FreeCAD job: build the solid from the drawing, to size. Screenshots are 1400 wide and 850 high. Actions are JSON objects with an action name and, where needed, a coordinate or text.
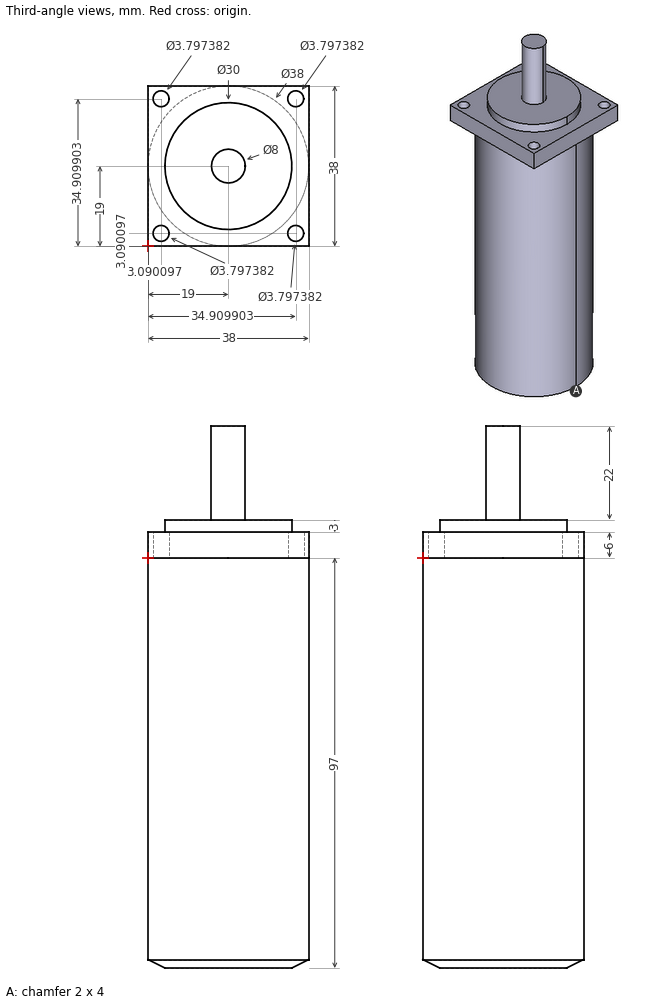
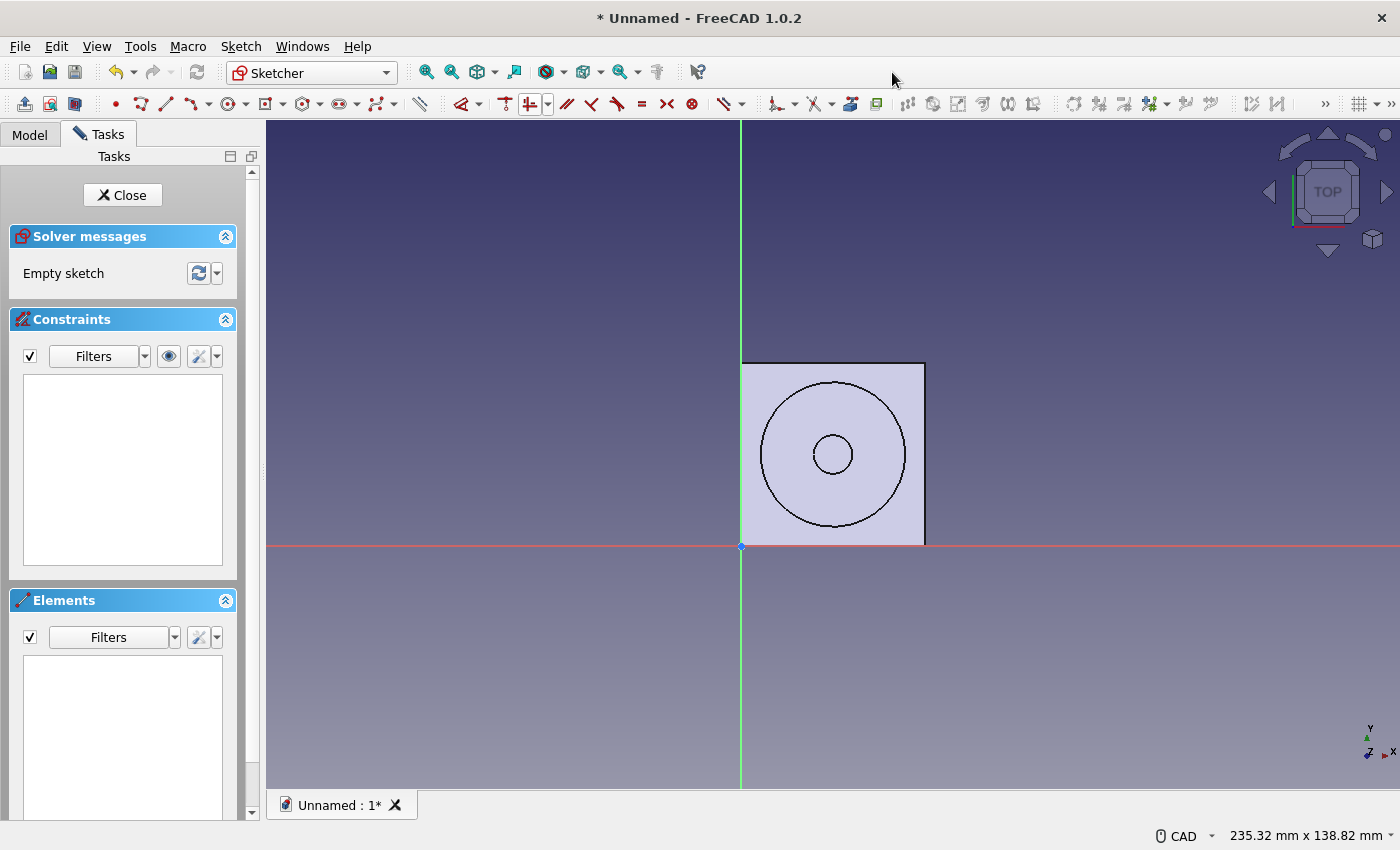
{"action": "scroll", "coordinate": [756, 374], "scroll_direction": "up", "scroll_amount": 15}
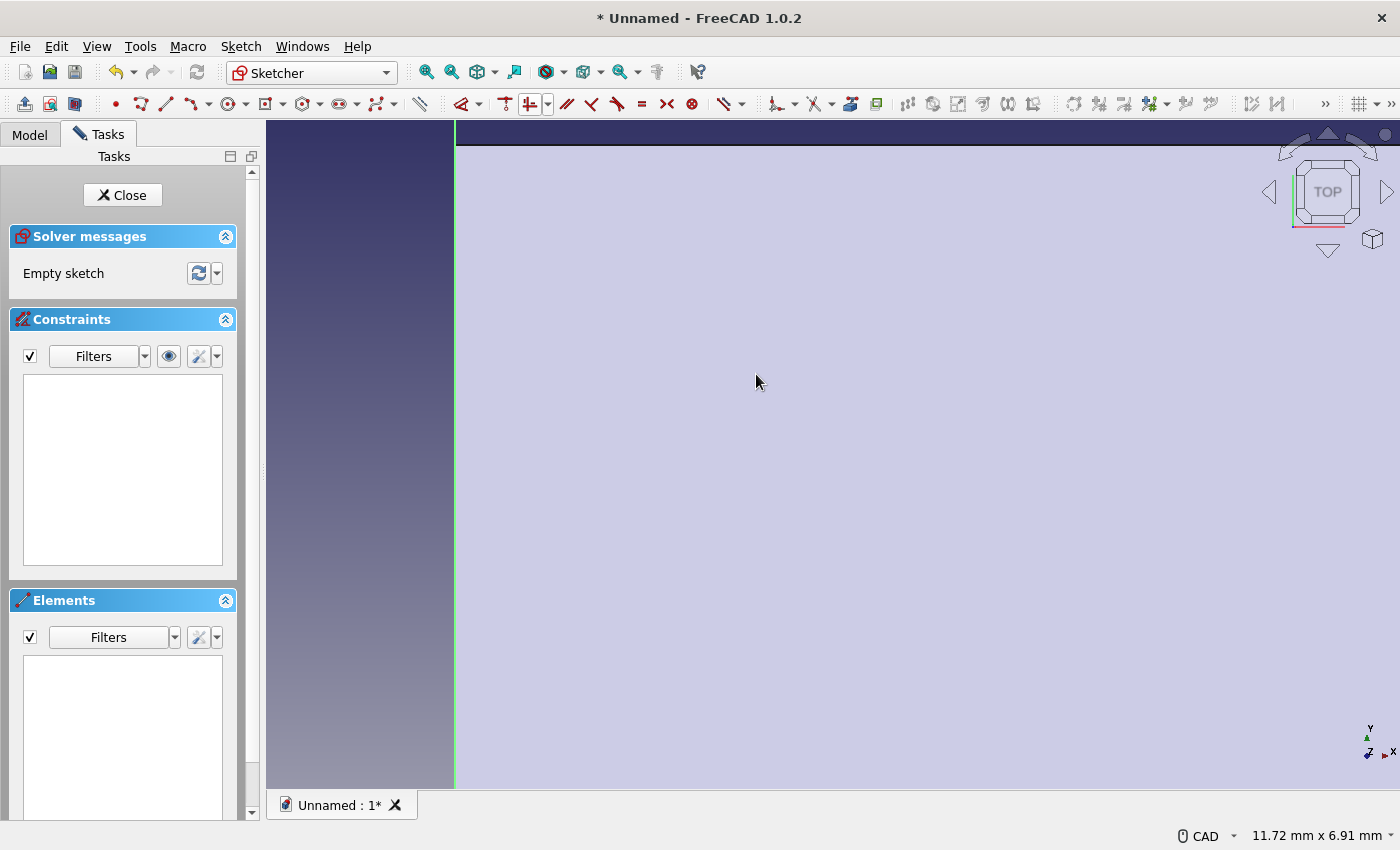
{"action": "key", "text": "g c"}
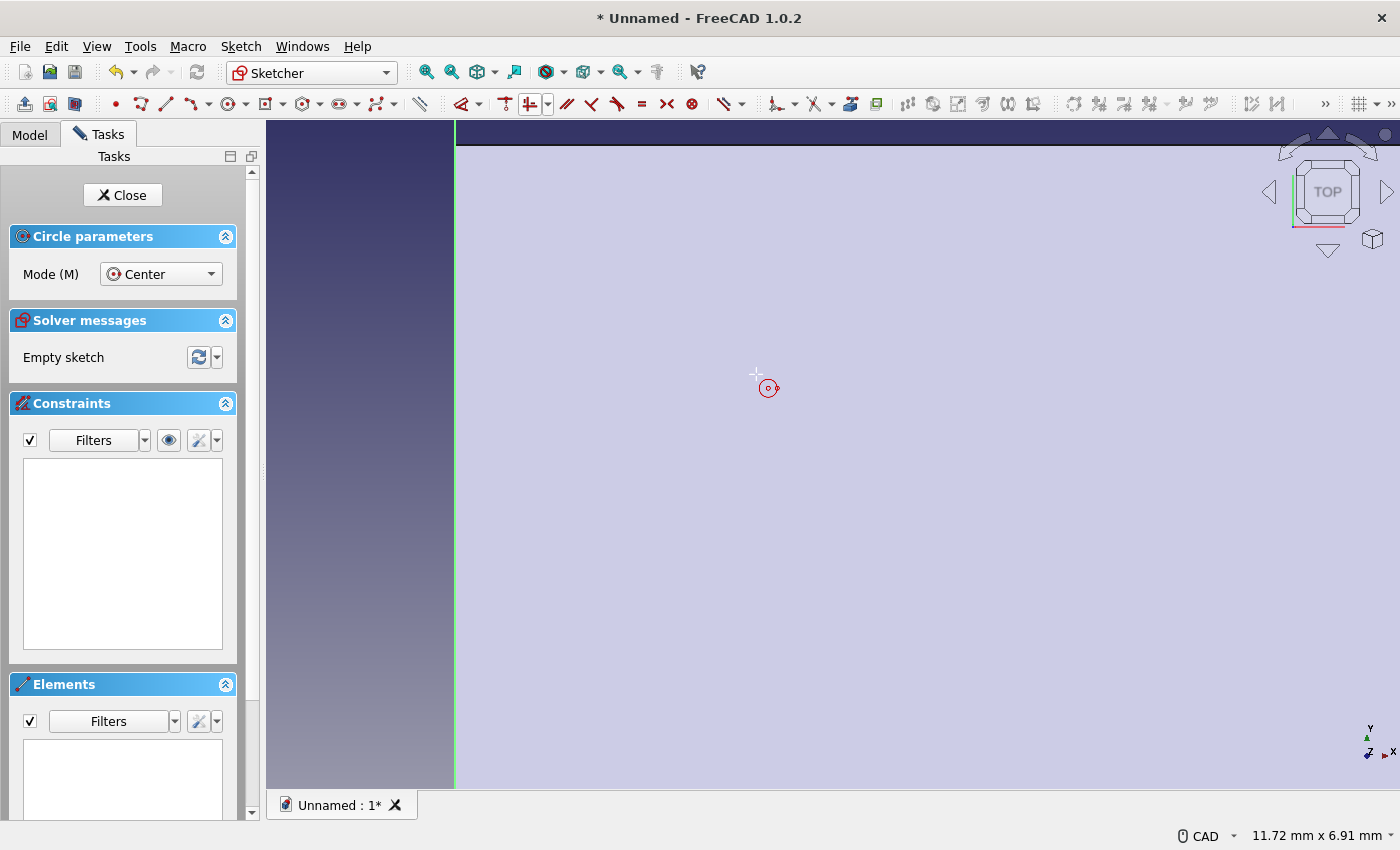
{"action": "left_click", "coordinate": [754, 444]}
{"action": "mouse_move", "coordinate": [884, 314]}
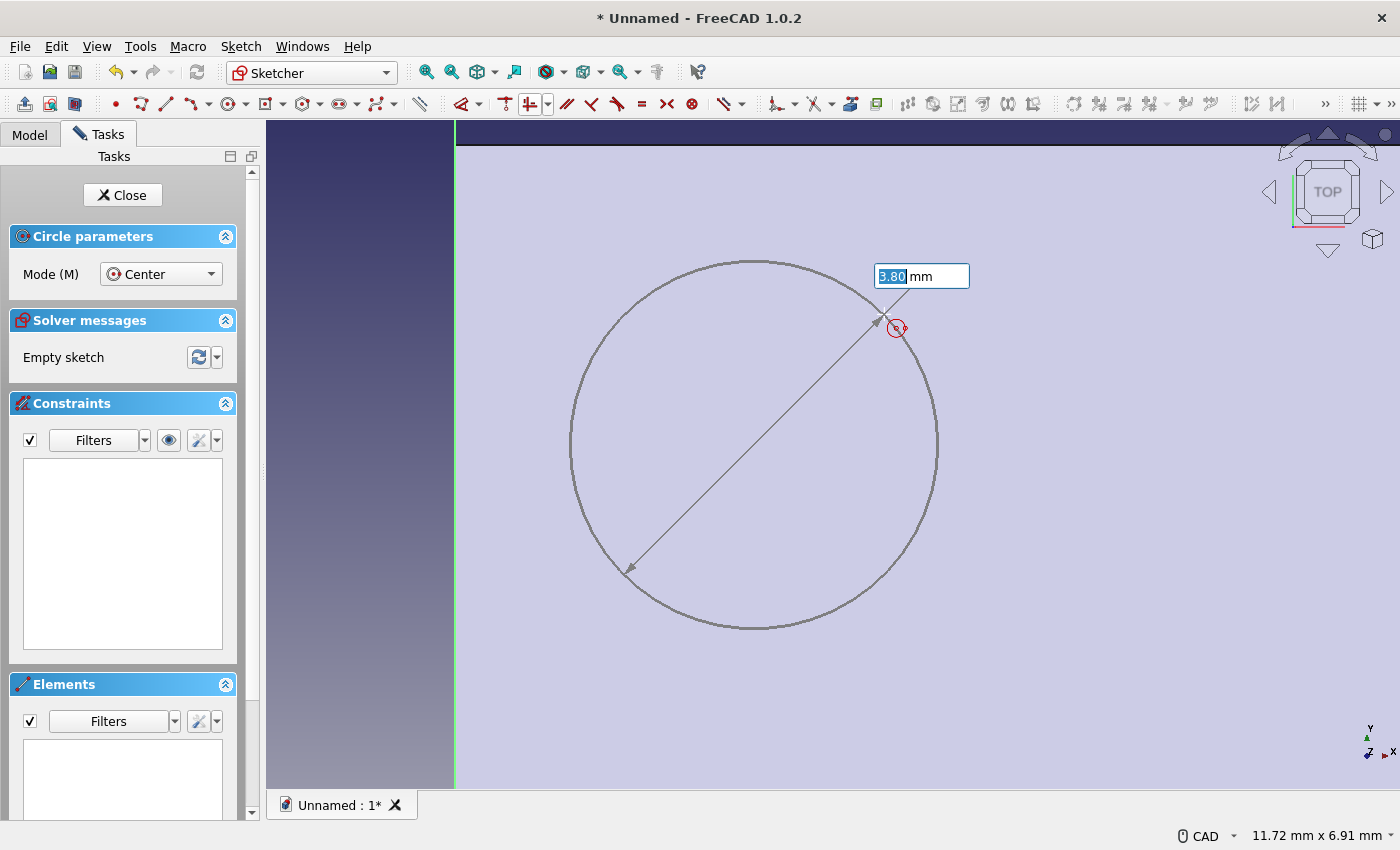
{"action": "type", "text": "3.797382"}
{"action": "key", "text": "Return"}
{"action": "key", "text": "Escape"}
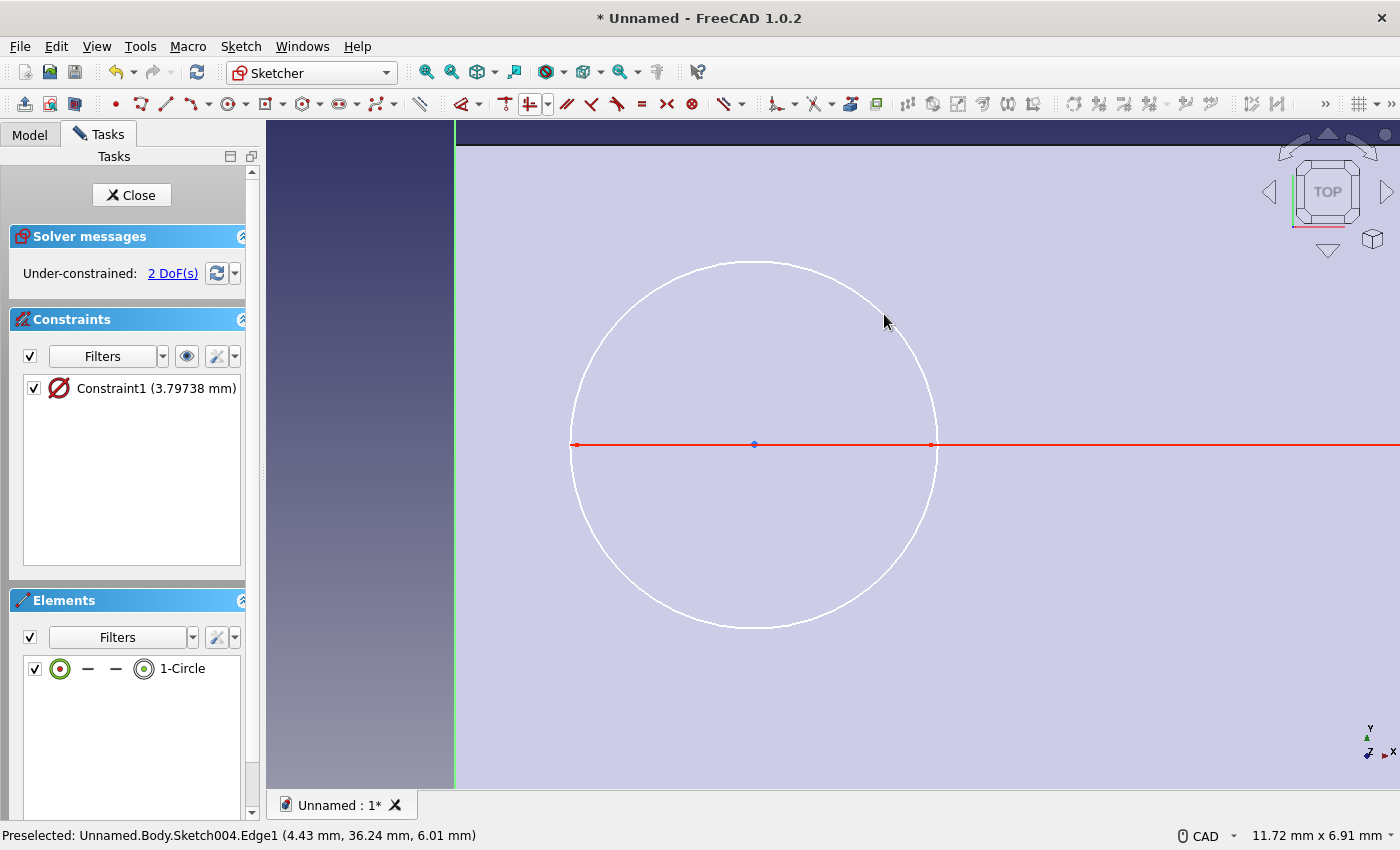
{"action": "key", "text": "d"}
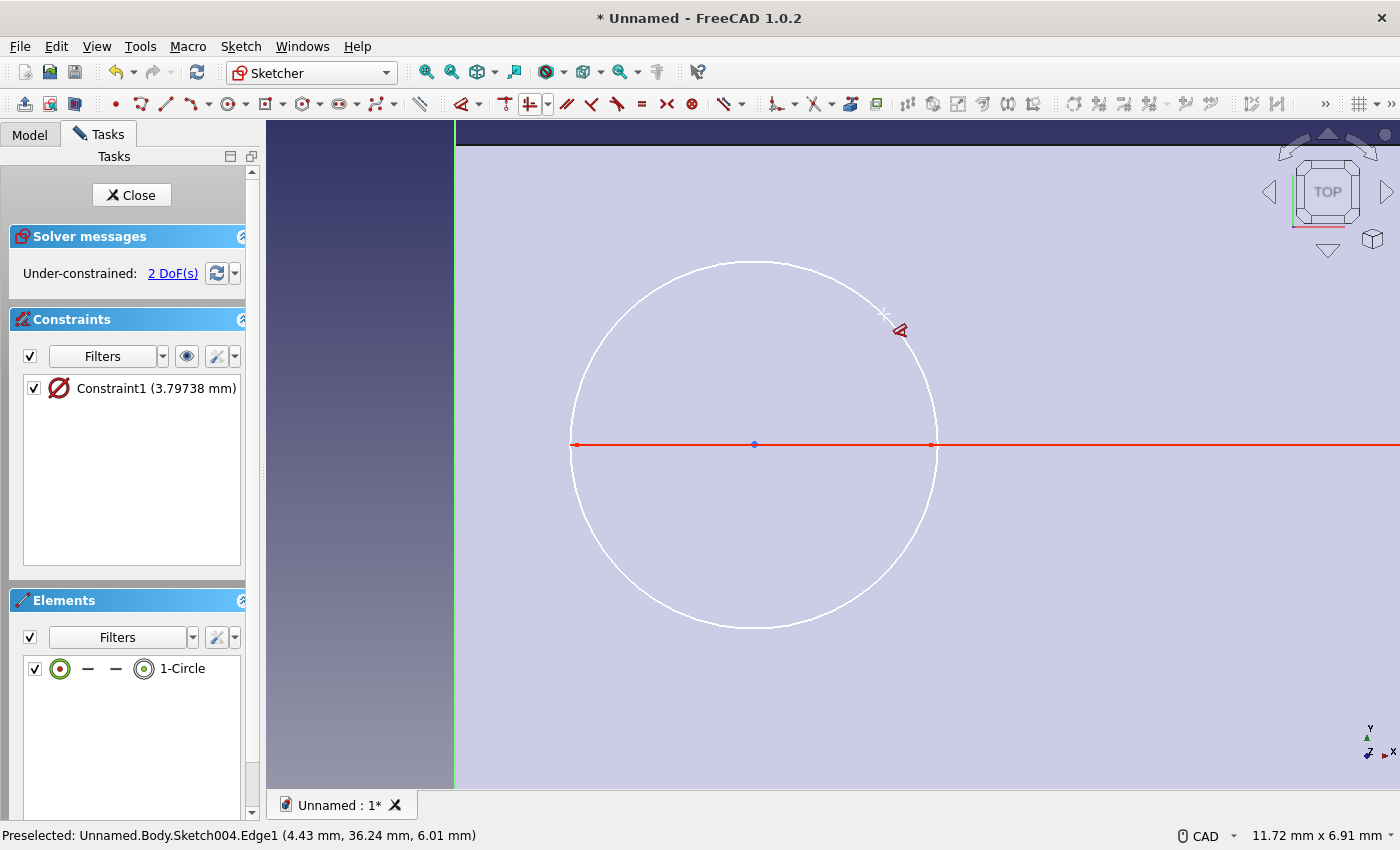
{"action": "left_click", "coordinate": [754, 445]}
{"action": "left_click", "coordinate": [605, 411]}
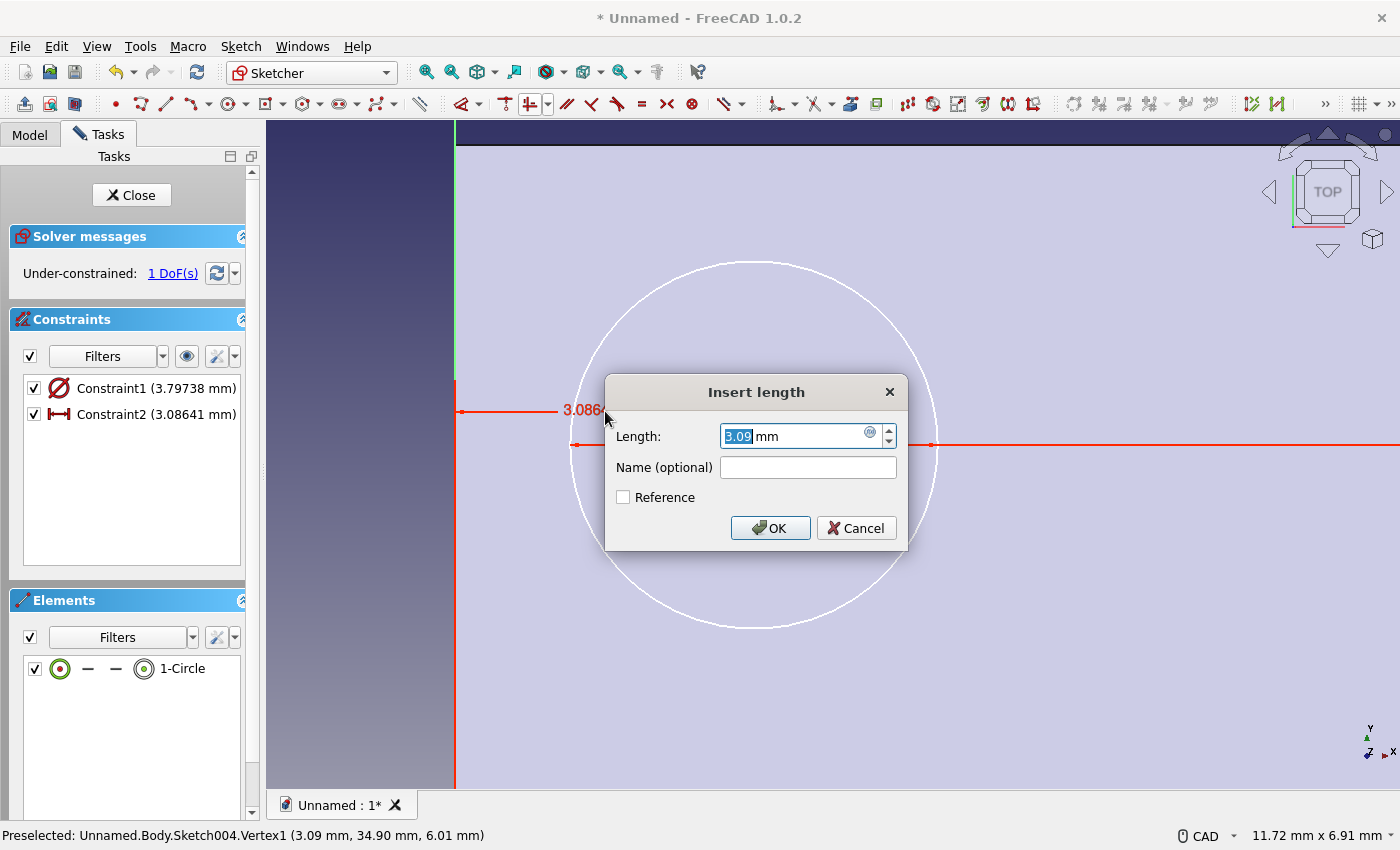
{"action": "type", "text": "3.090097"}
{"action": "key", "text": "Return"}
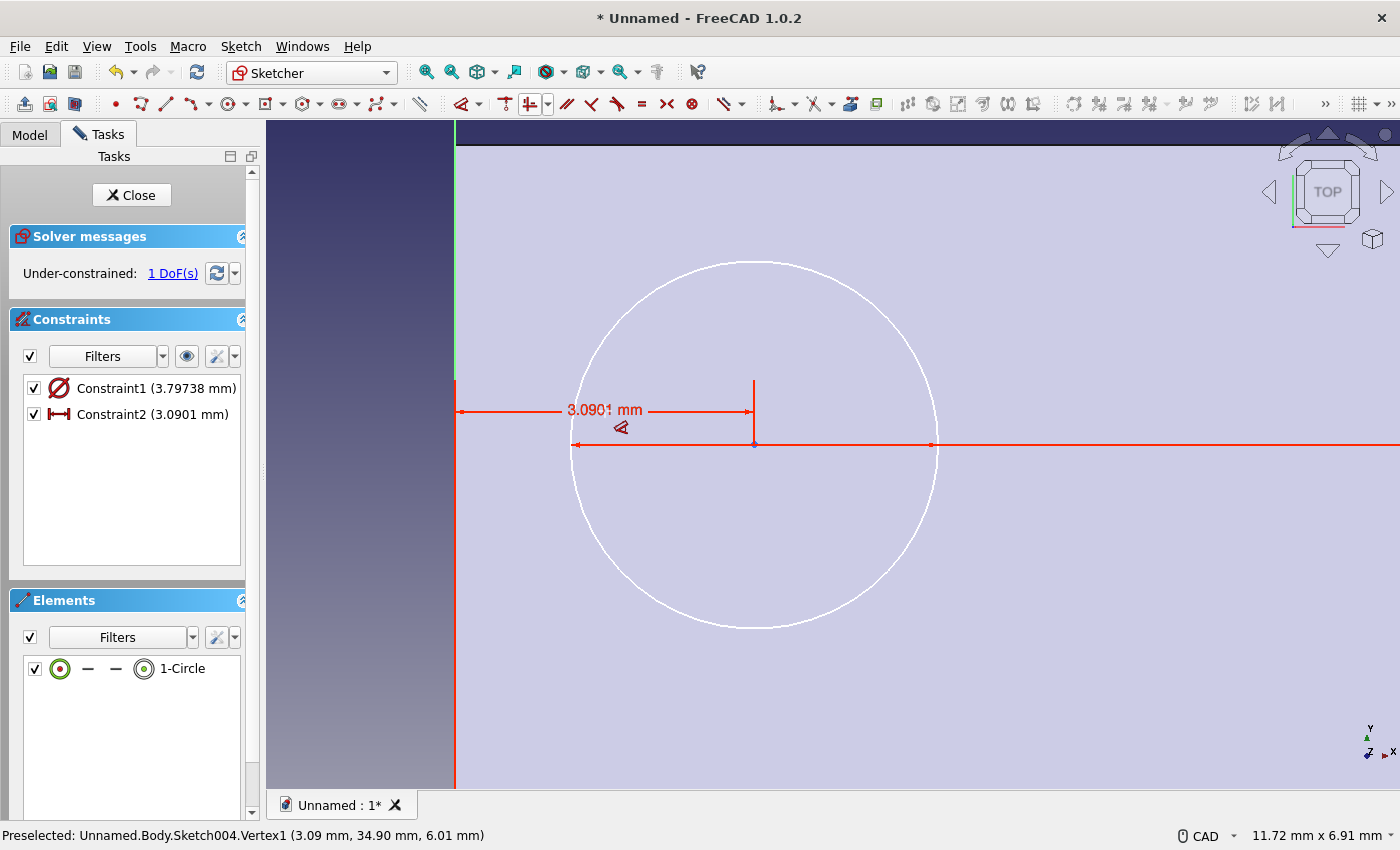
{"action": "left_click", "coordinate": [754, 445]}
{"action": "left_click", "coordinate": [421, 603]}